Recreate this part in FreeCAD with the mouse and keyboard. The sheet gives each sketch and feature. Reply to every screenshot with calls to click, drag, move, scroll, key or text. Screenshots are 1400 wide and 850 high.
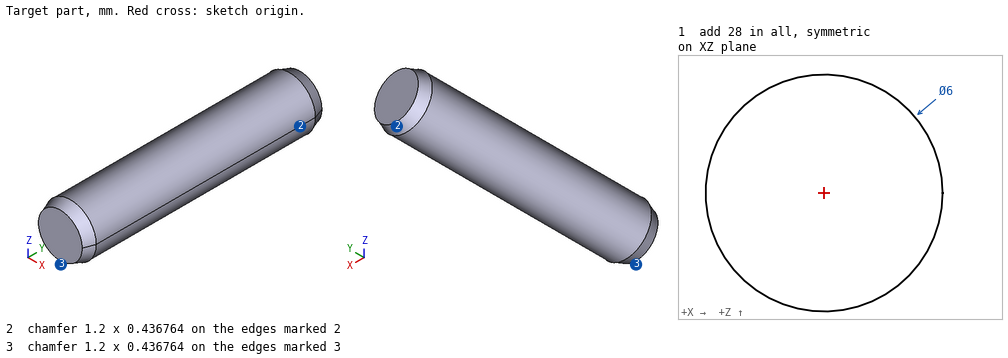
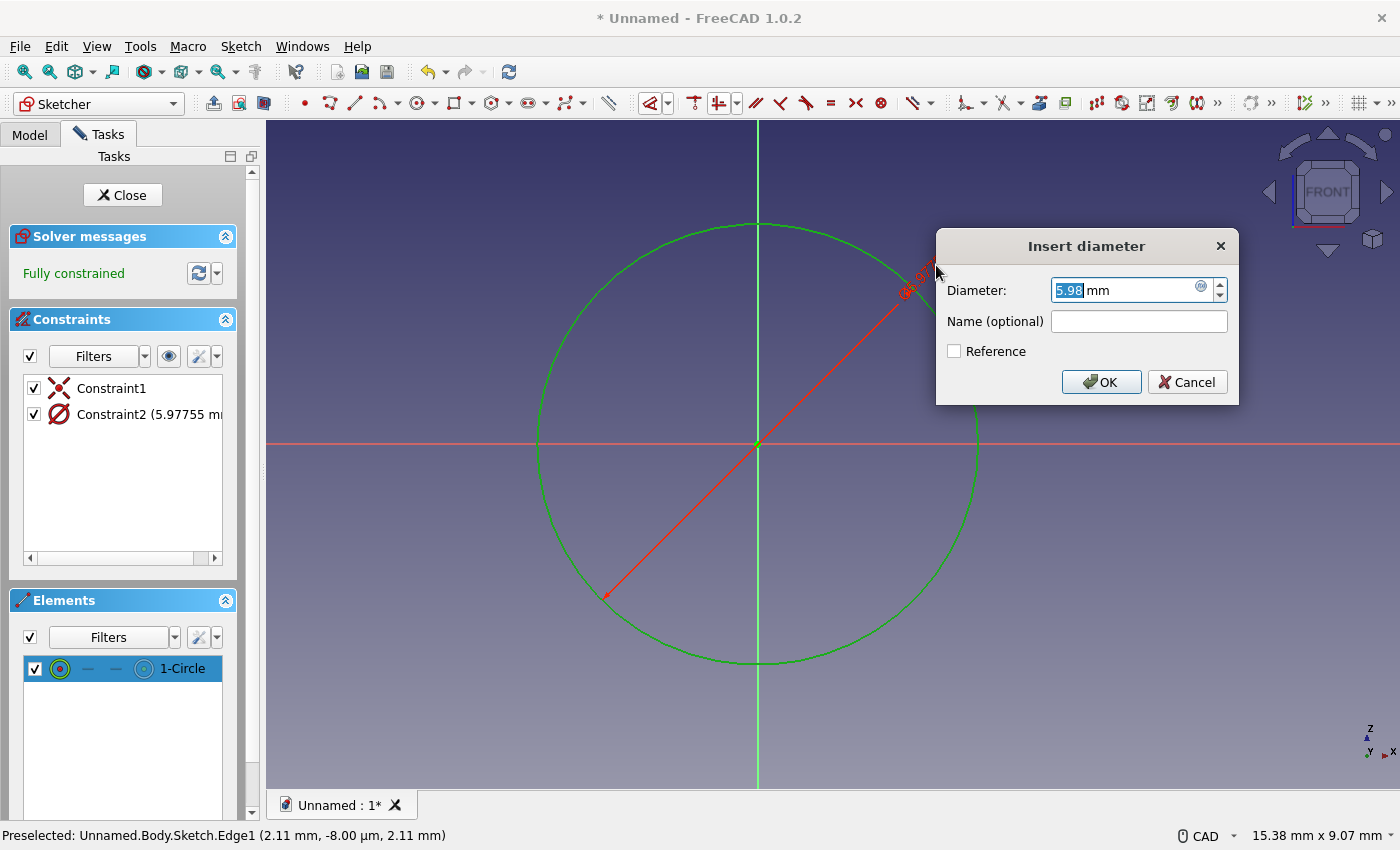
text(6)
key(Return)
key(Escape)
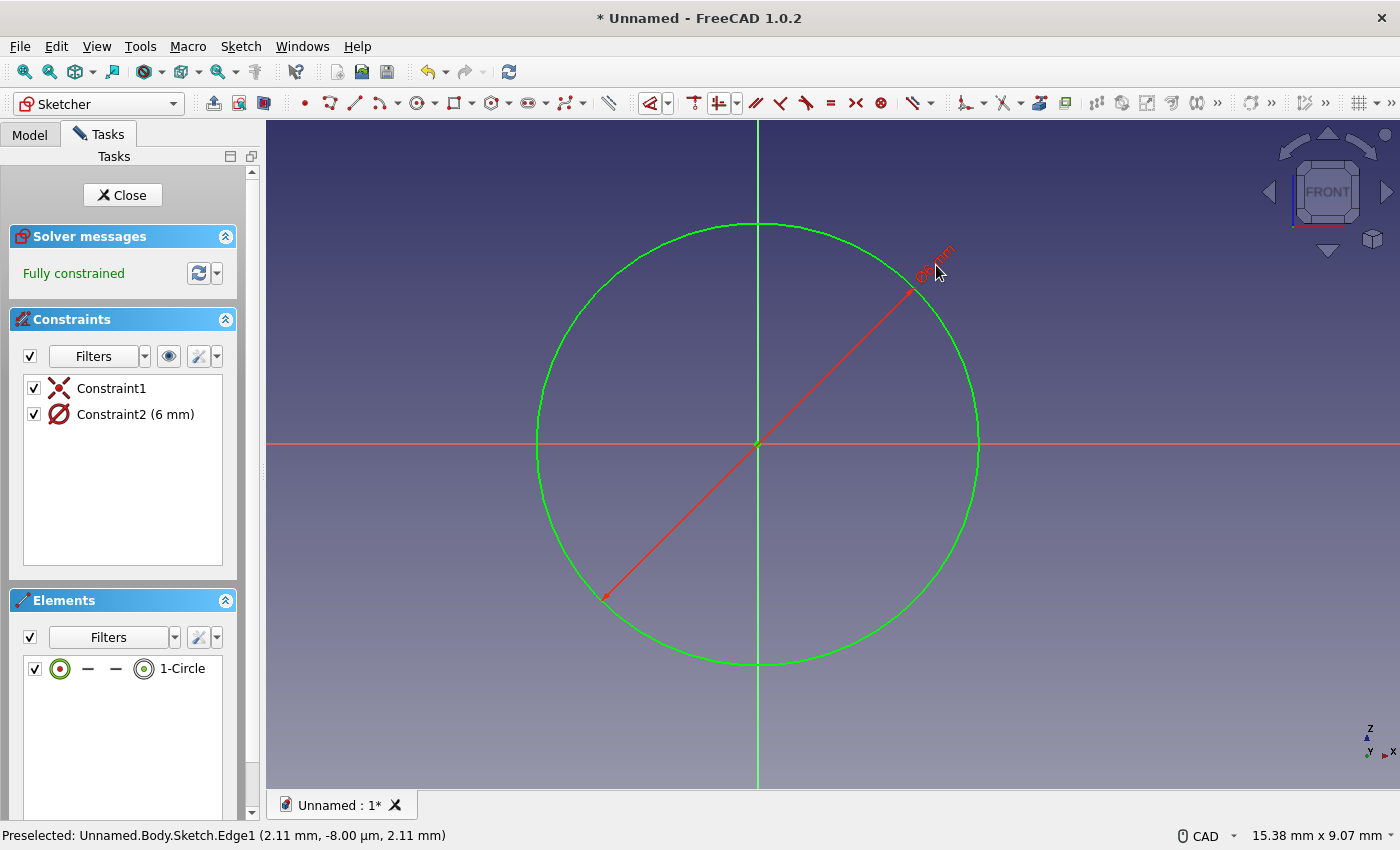
click(123, 195)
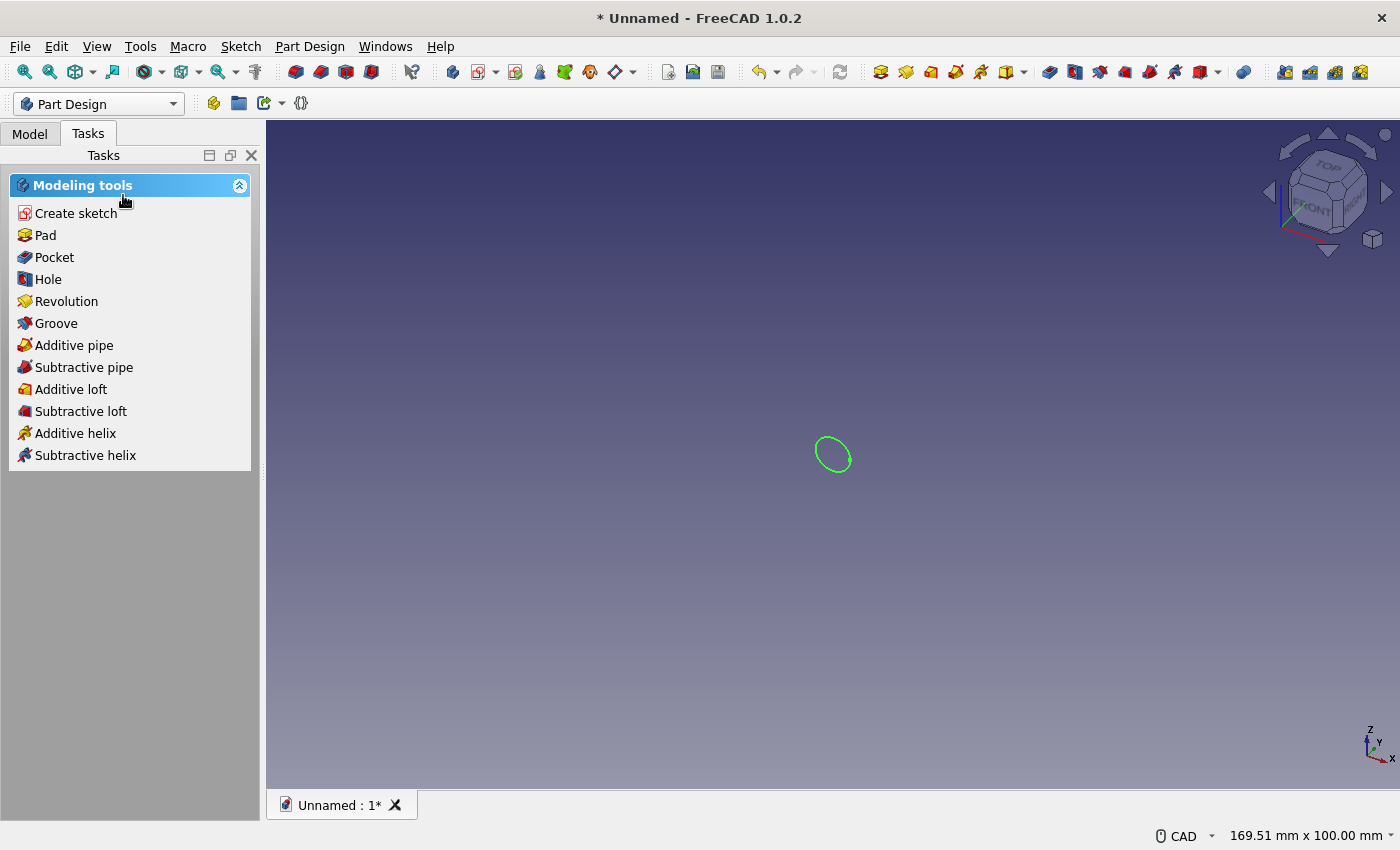
click(881, 72)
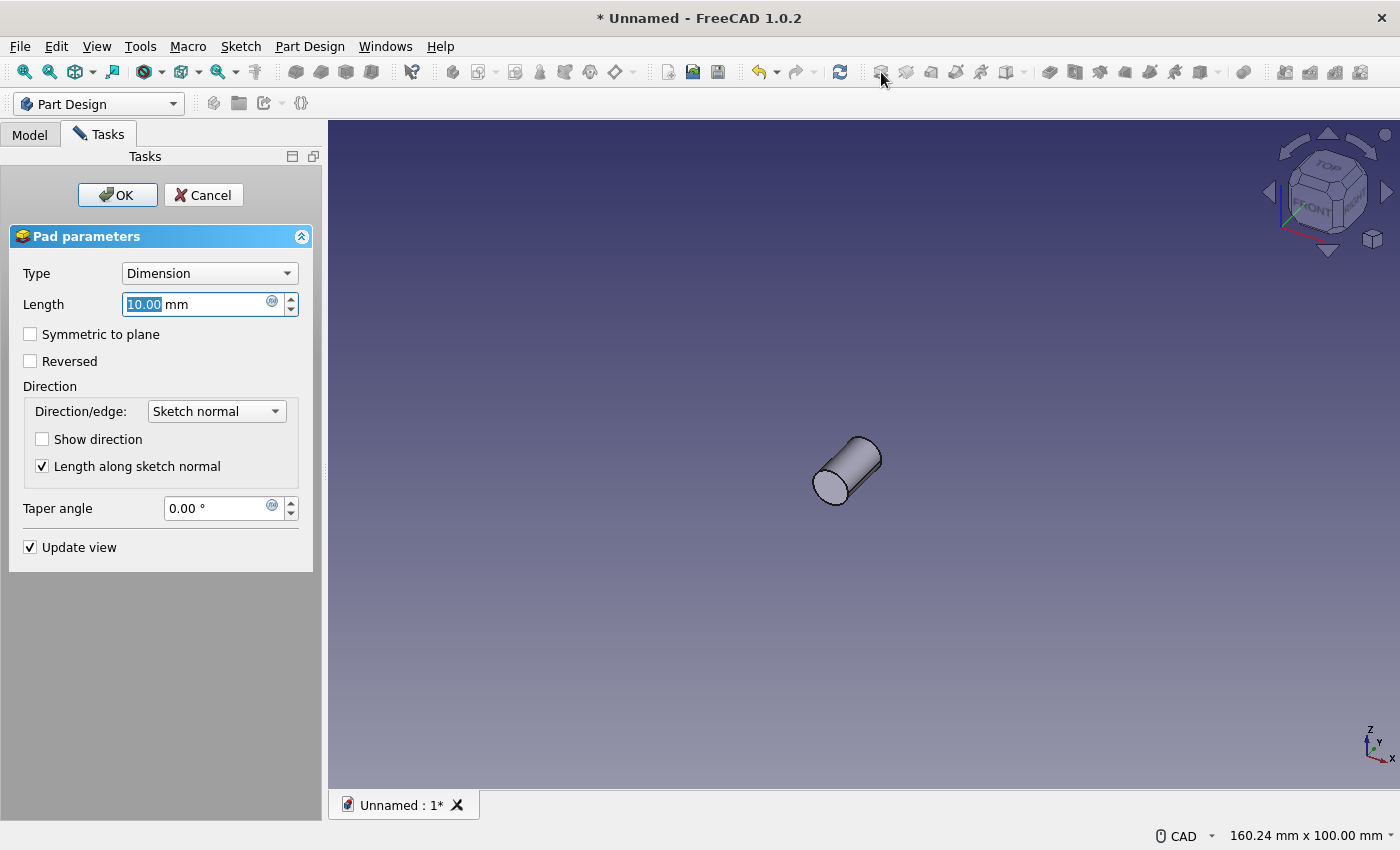
text(28)
key(Tab)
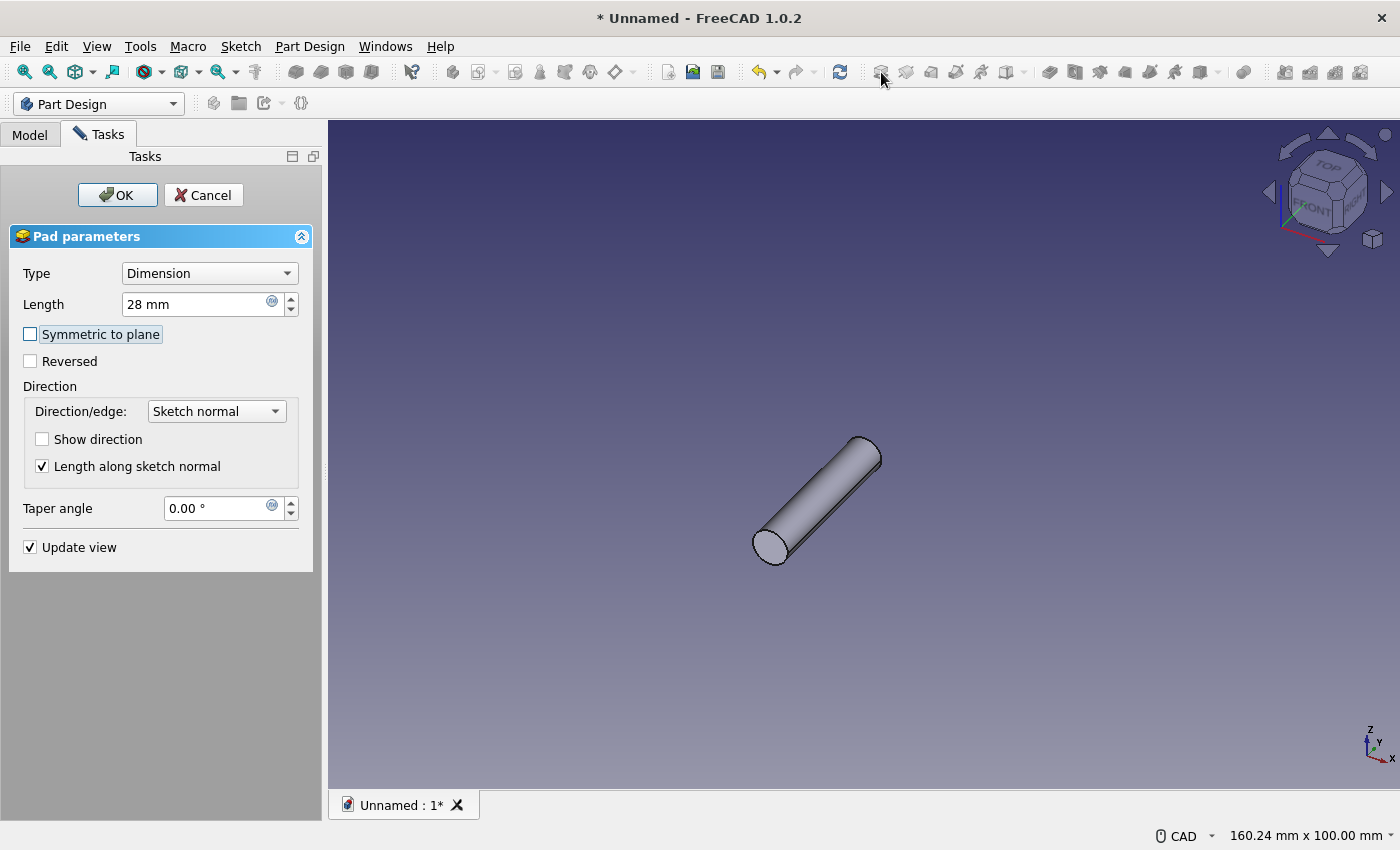
click(31, 334)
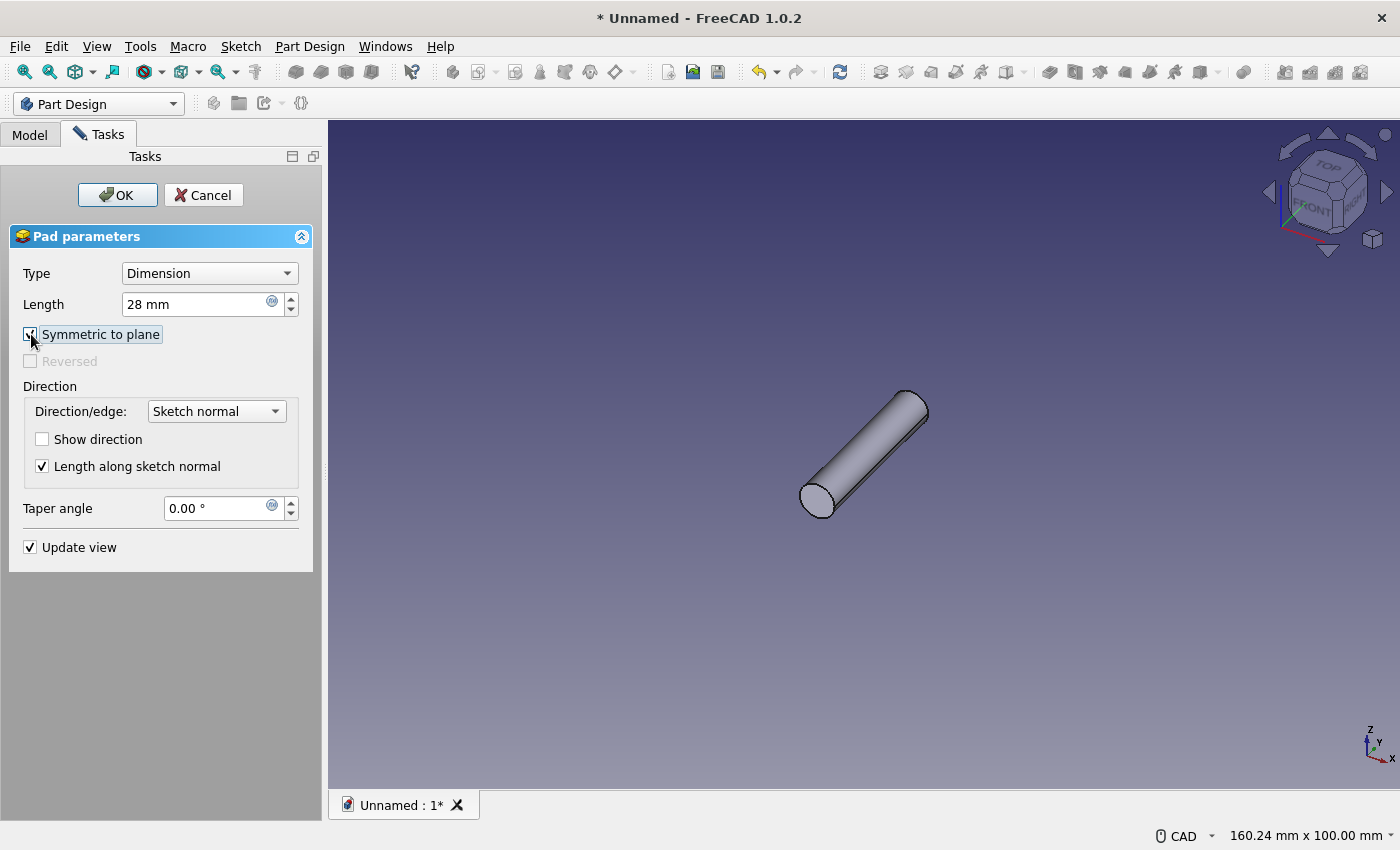
click(118, 195)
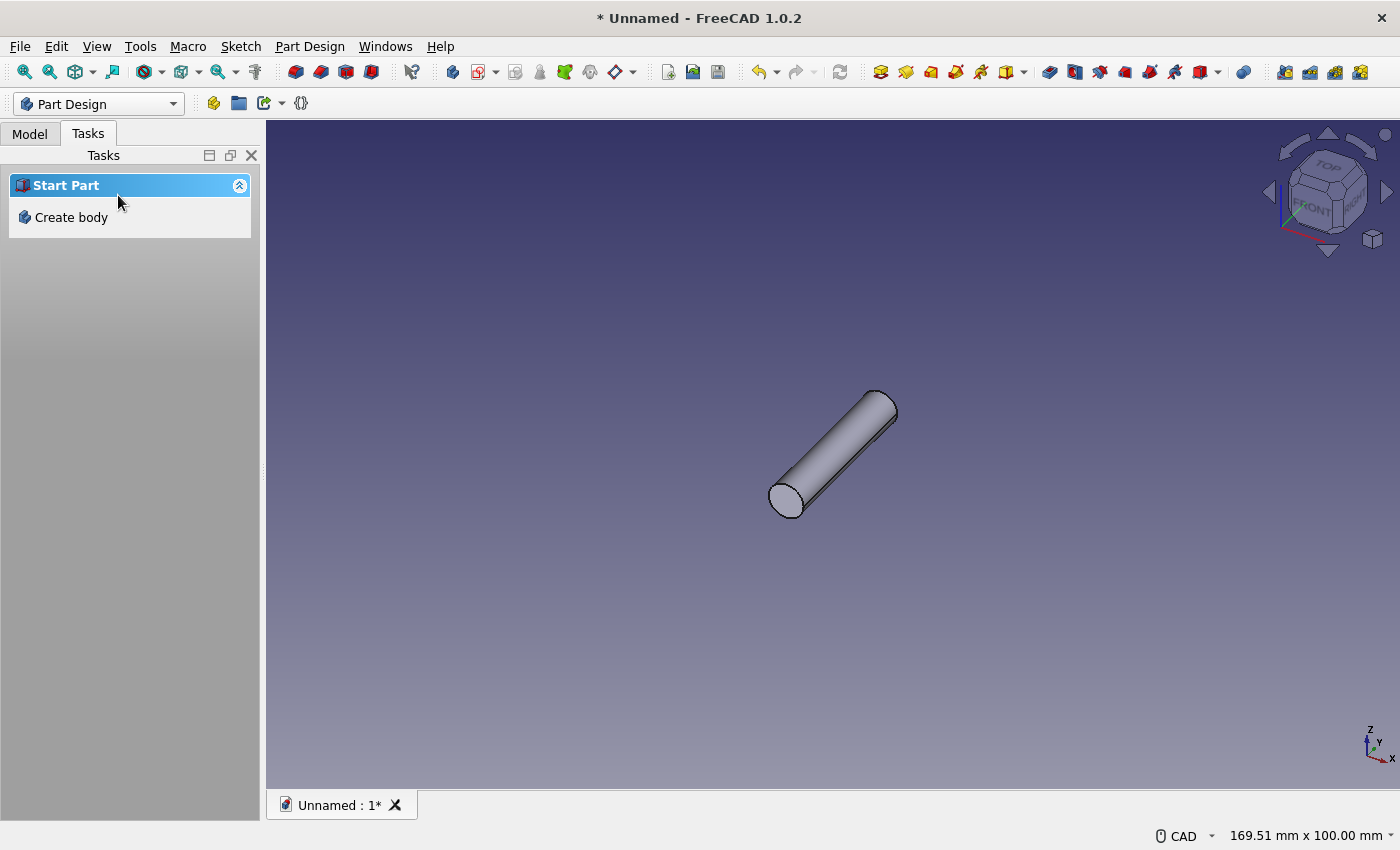
click(25, 72)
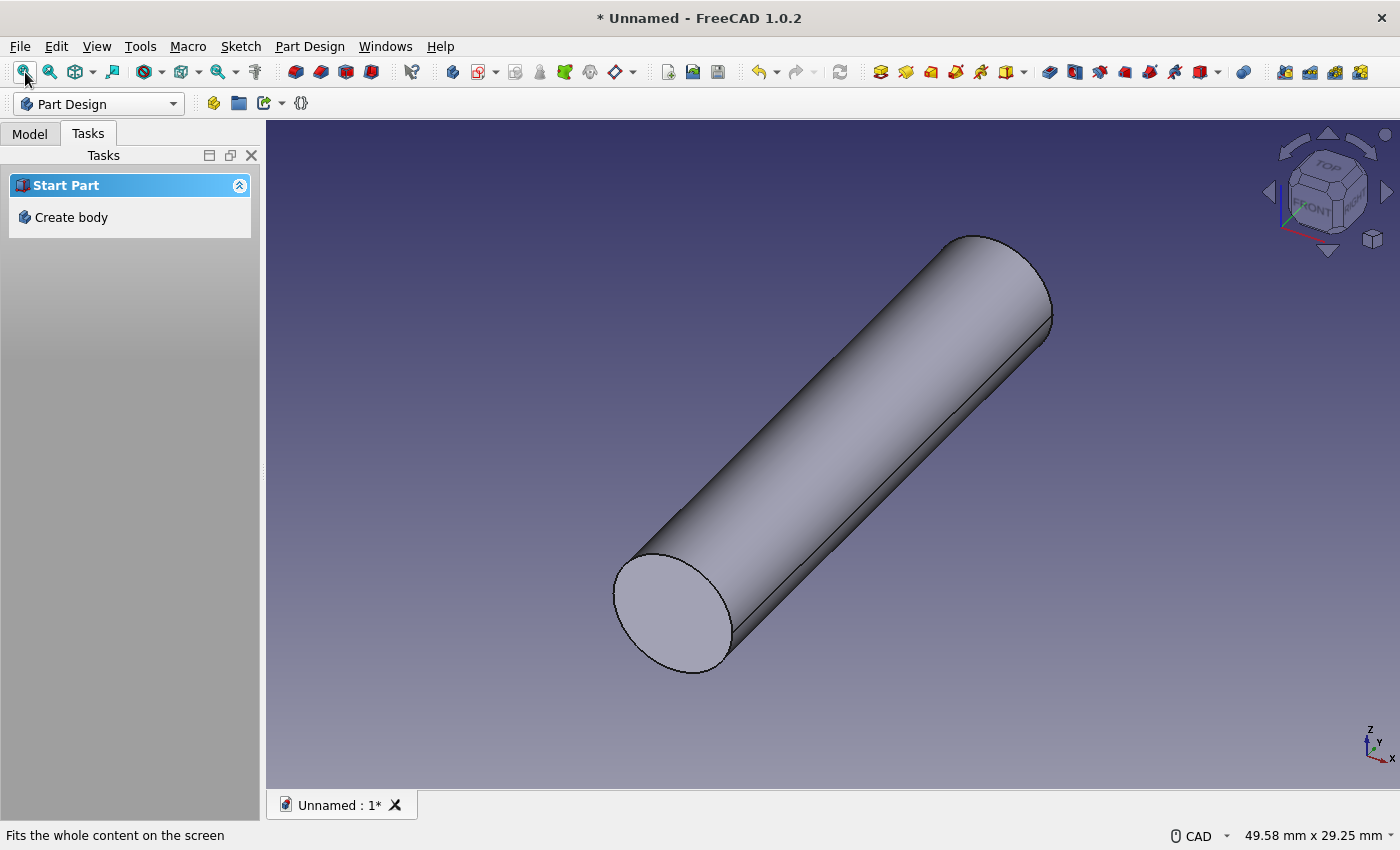
key(0)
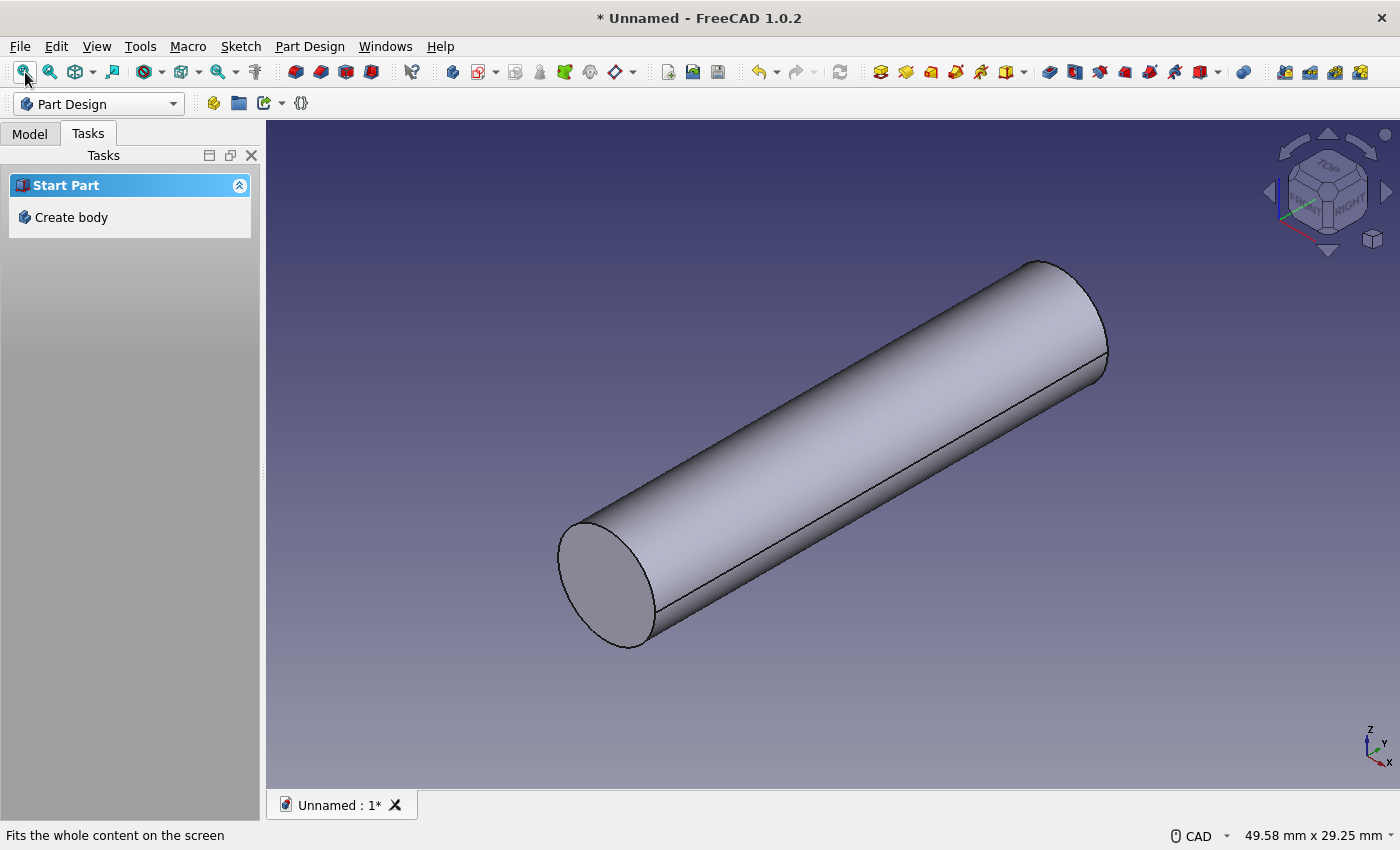
key(2)